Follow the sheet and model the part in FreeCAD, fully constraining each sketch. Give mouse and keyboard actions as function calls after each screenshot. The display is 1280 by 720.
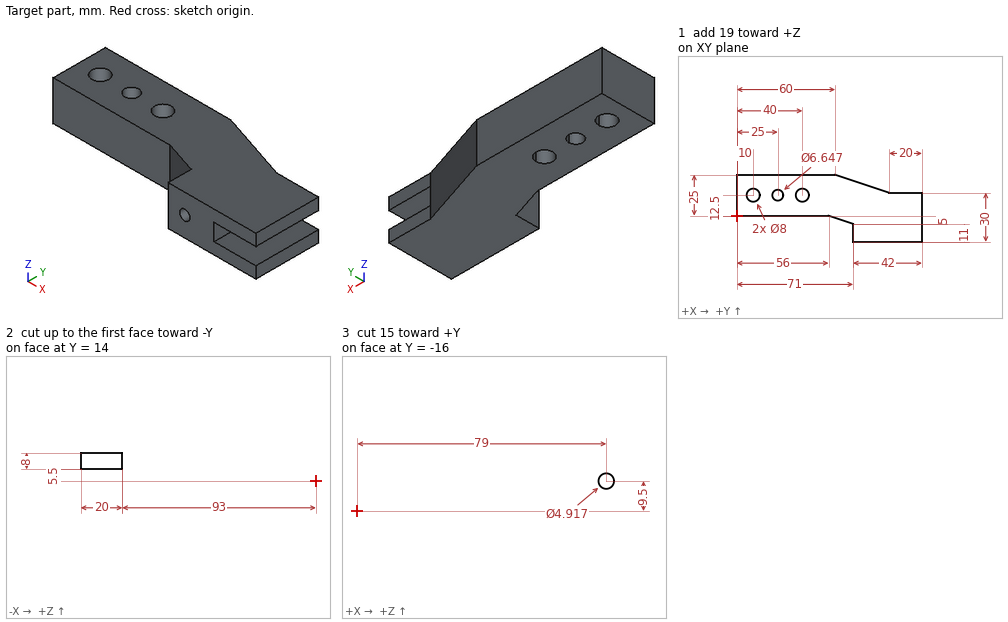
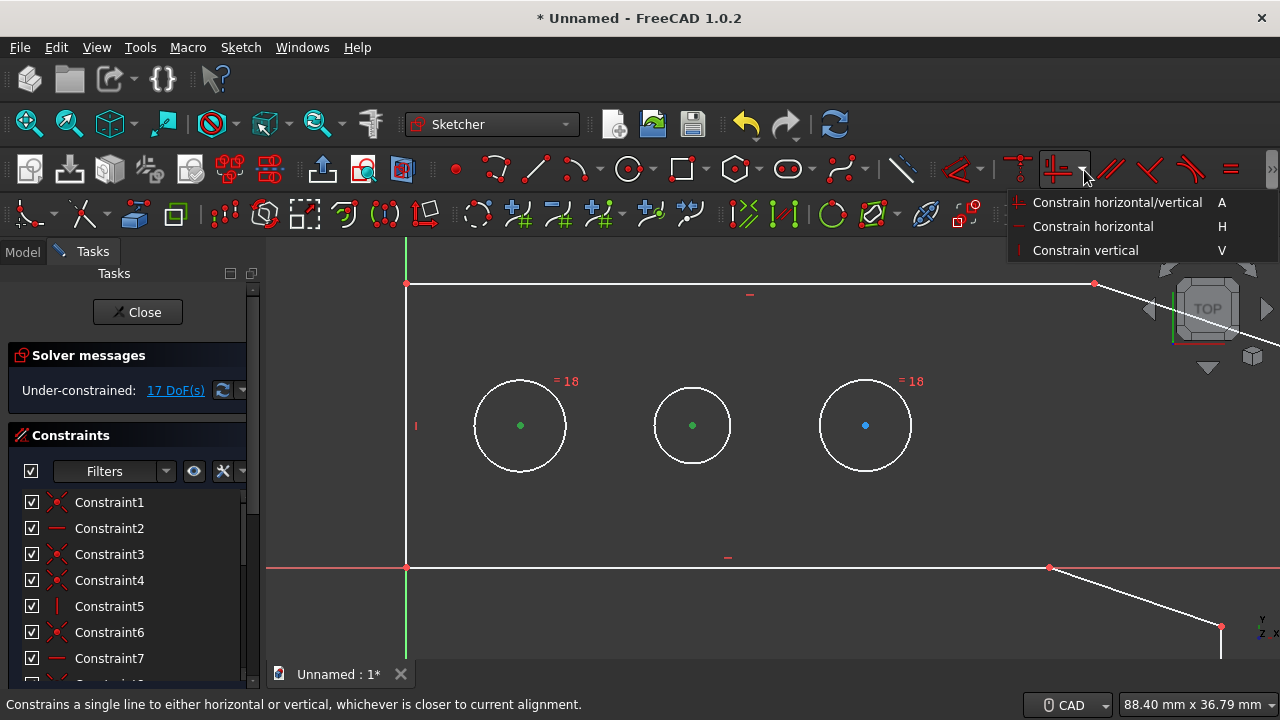
click(1143, 226)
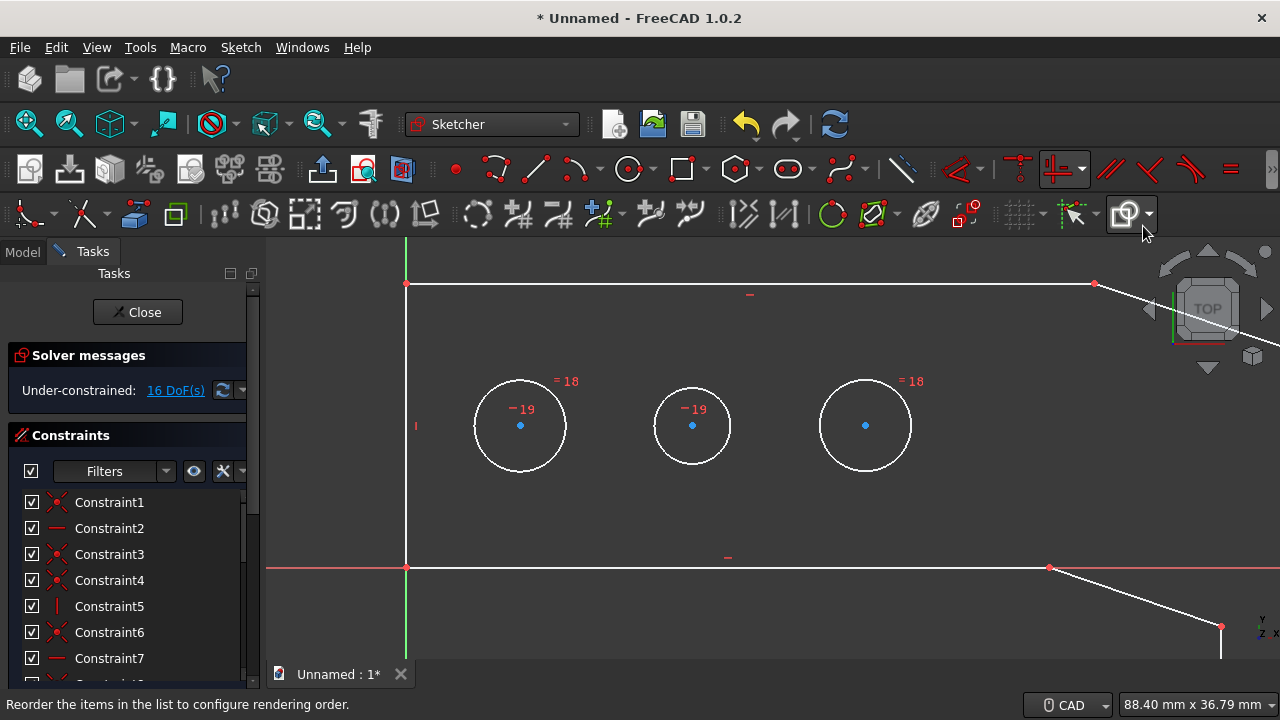
click(692, 426)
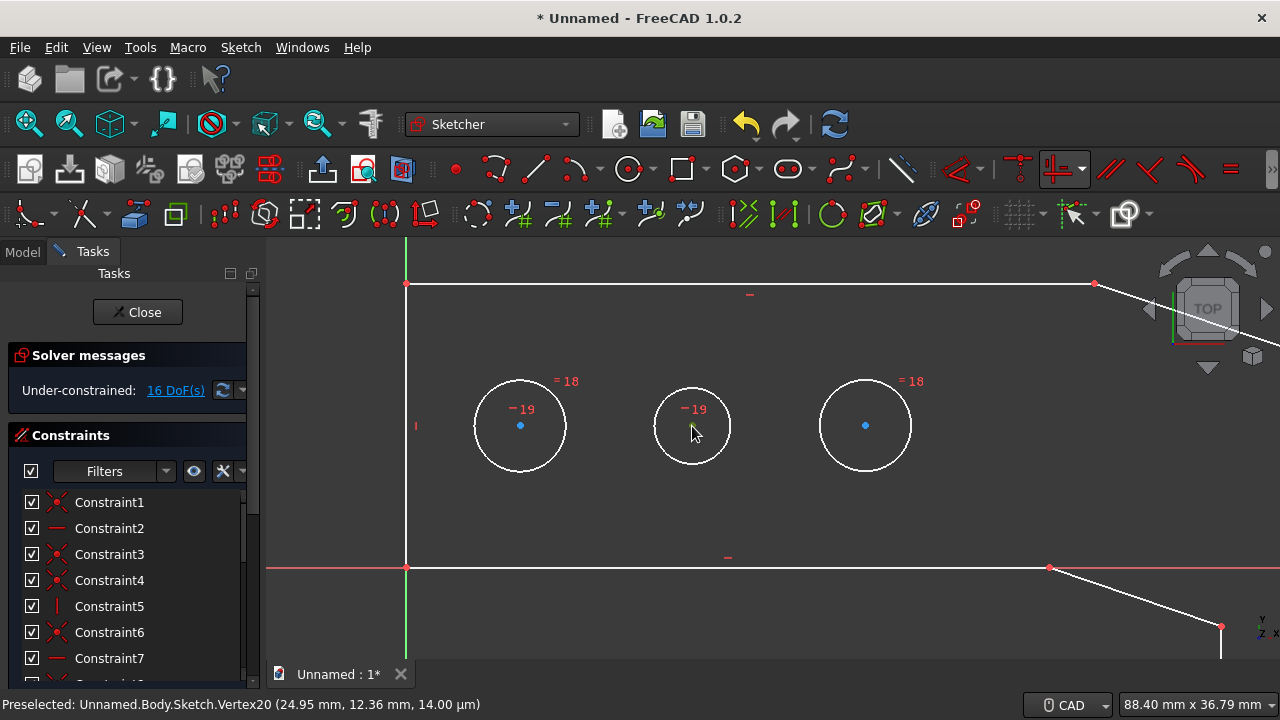
click(865, 426)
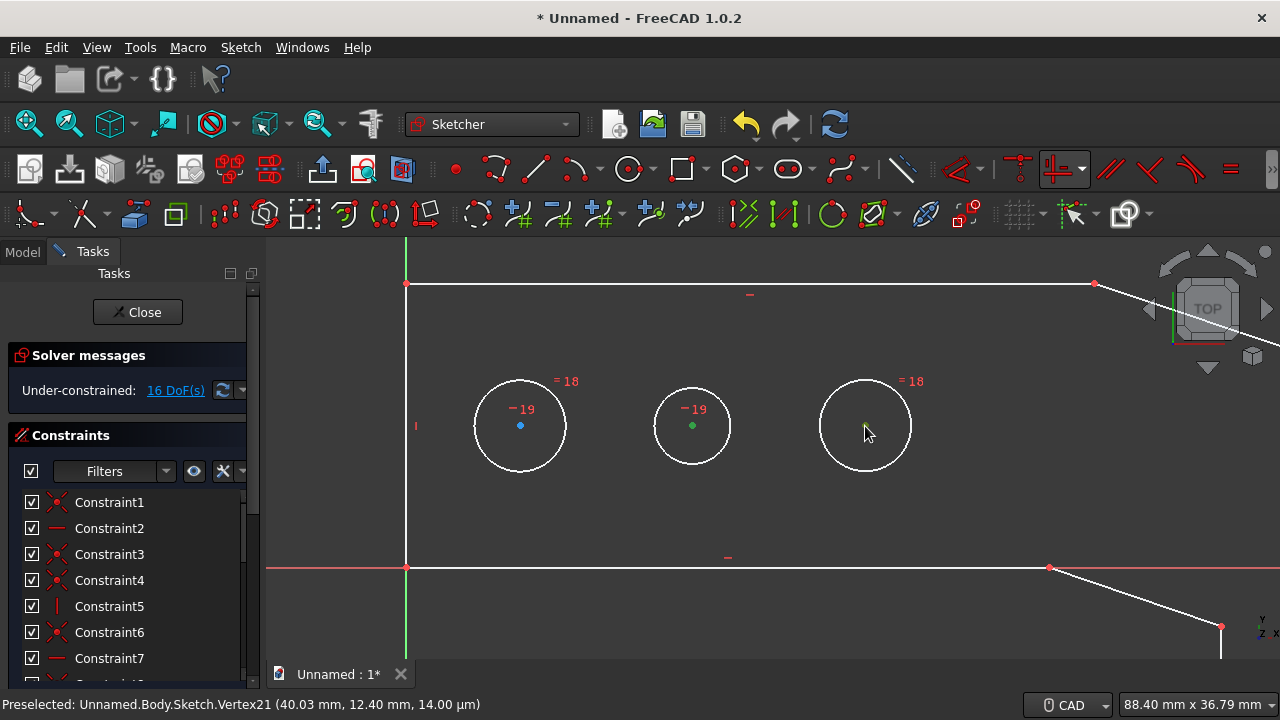
click(1084, 170)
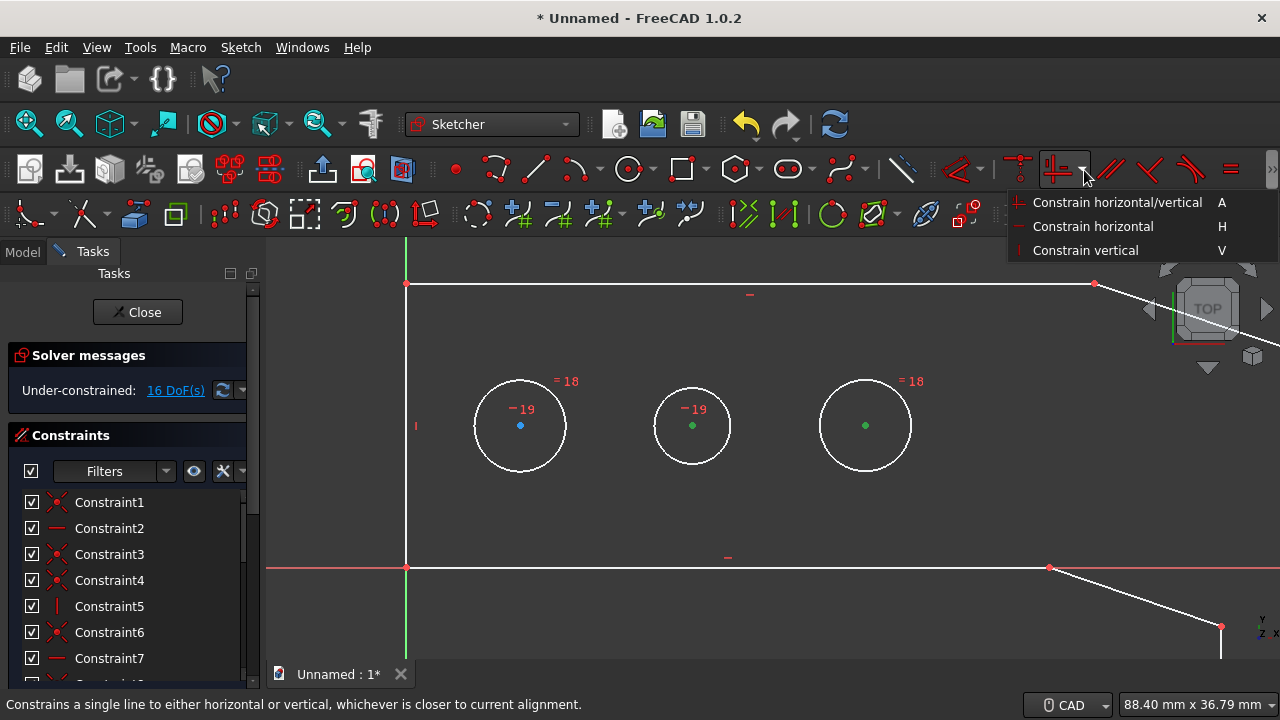
click(1143, 226)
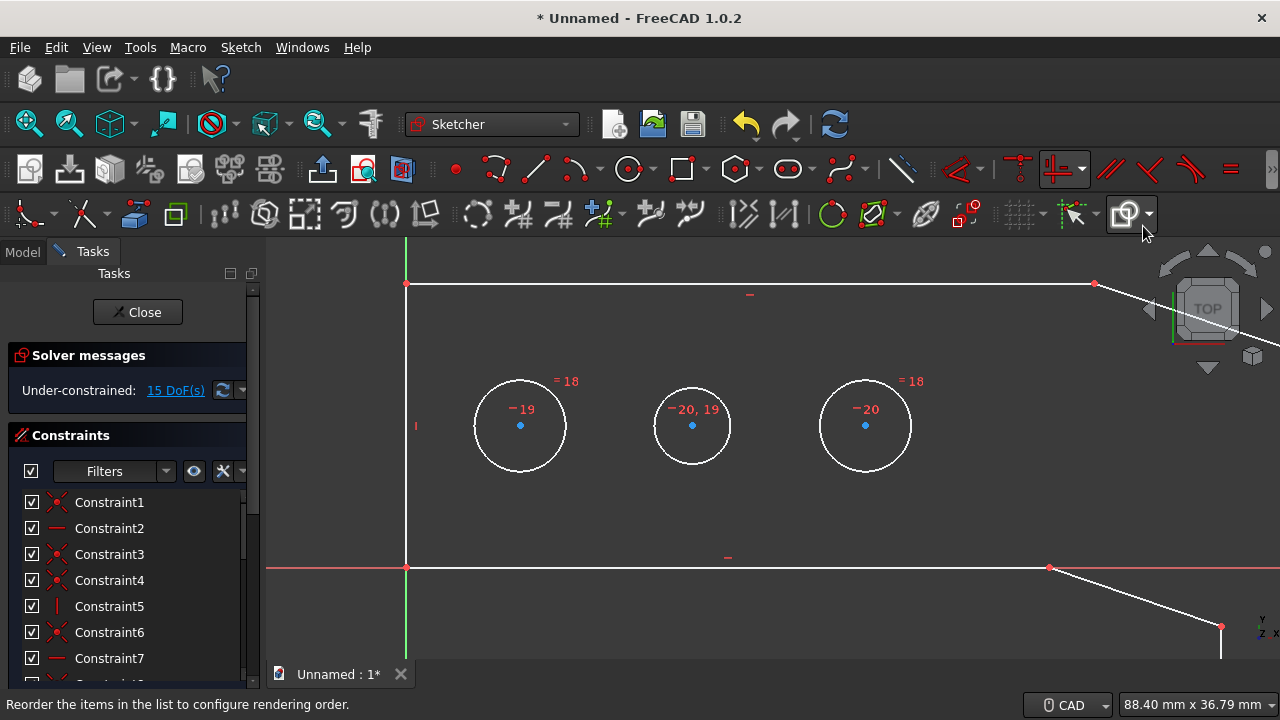
click(956, 170)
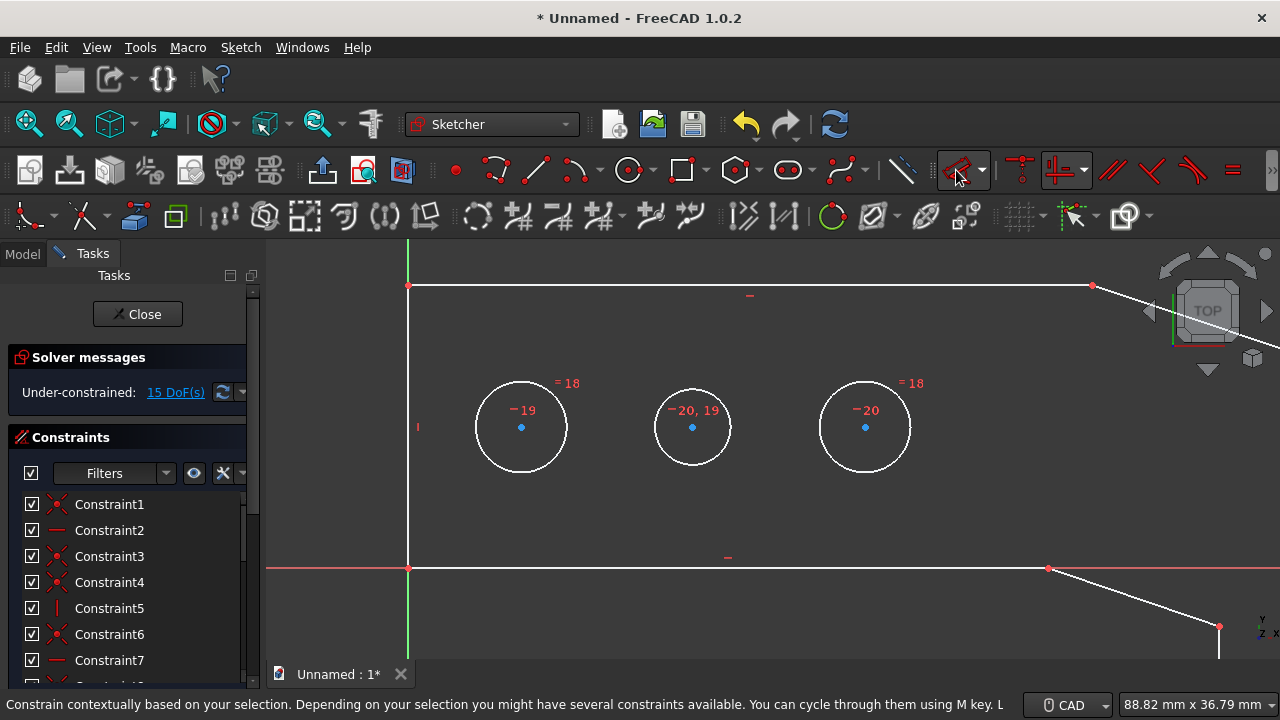
click(553, 395)
click(575, 372)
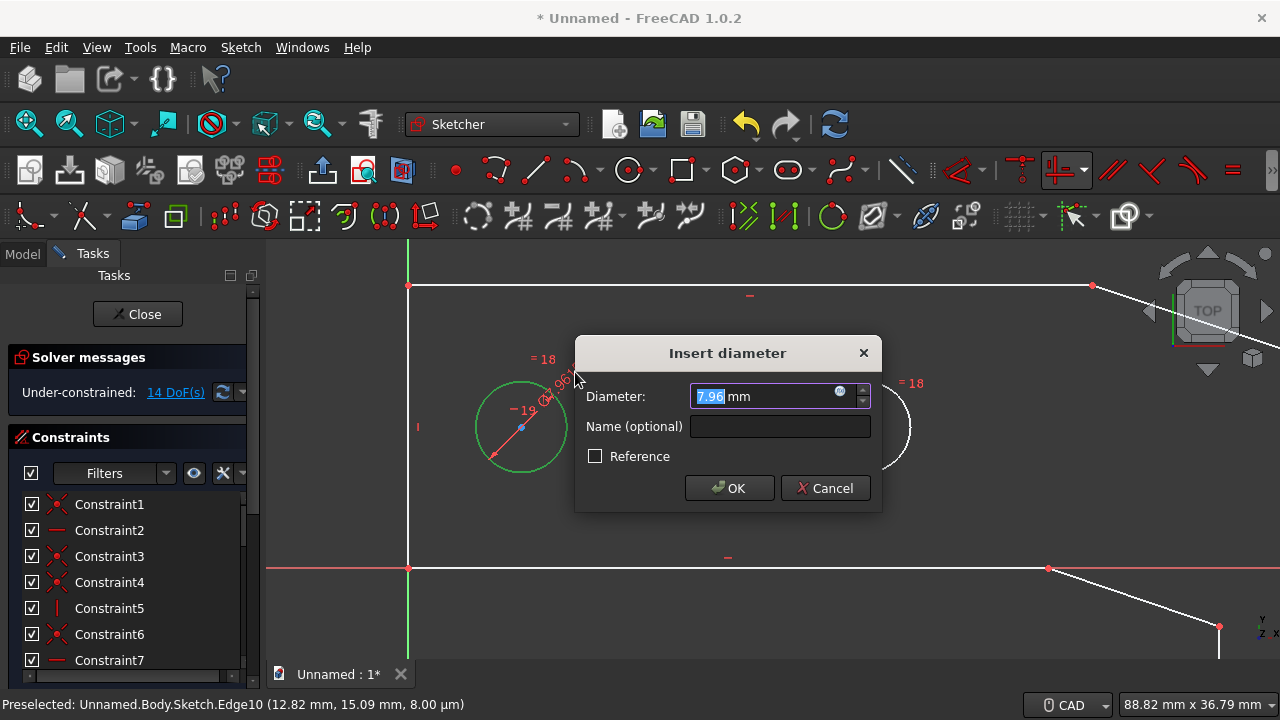
text(8)
key(Return)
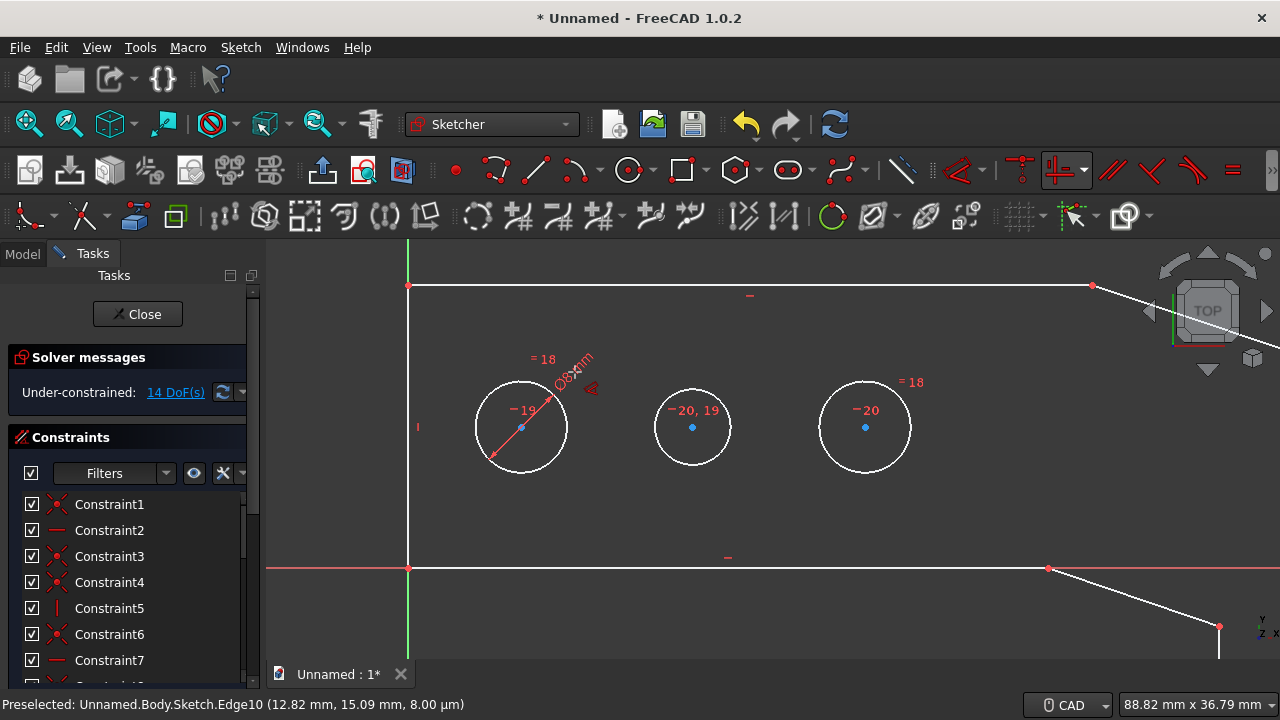
click(719, 400)
click(741, 377)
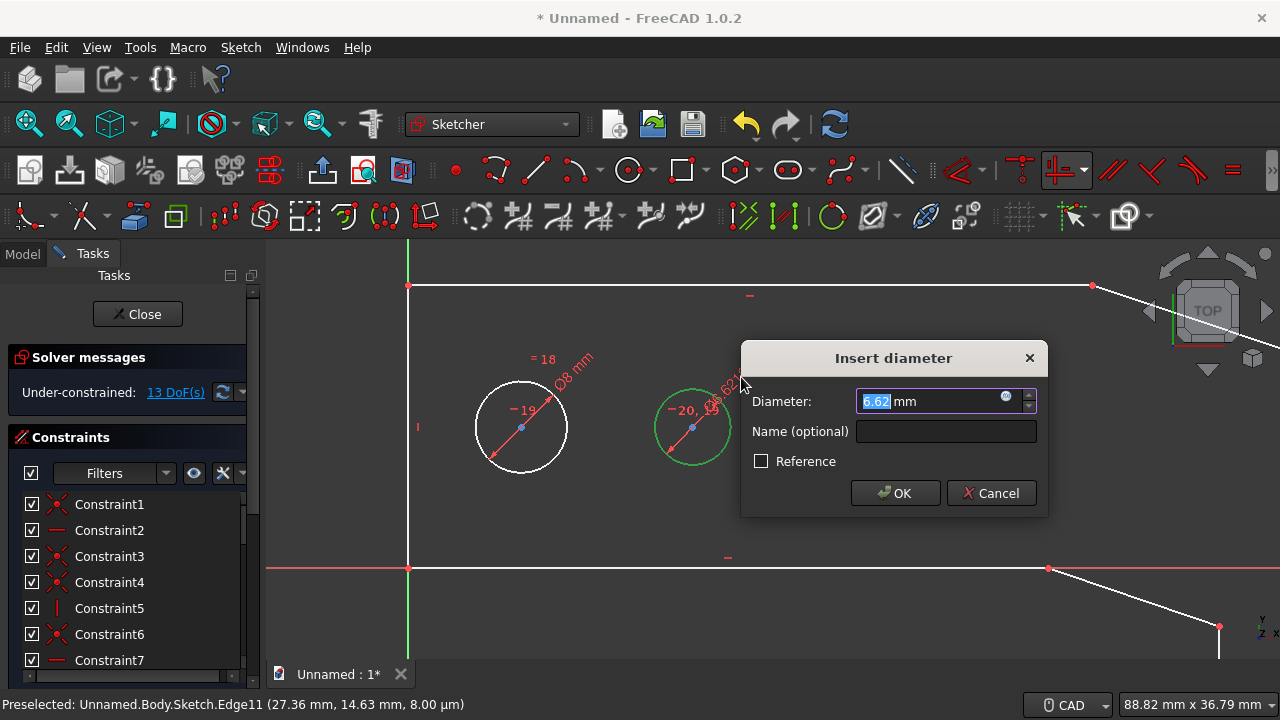
text(6.647)
key(Return)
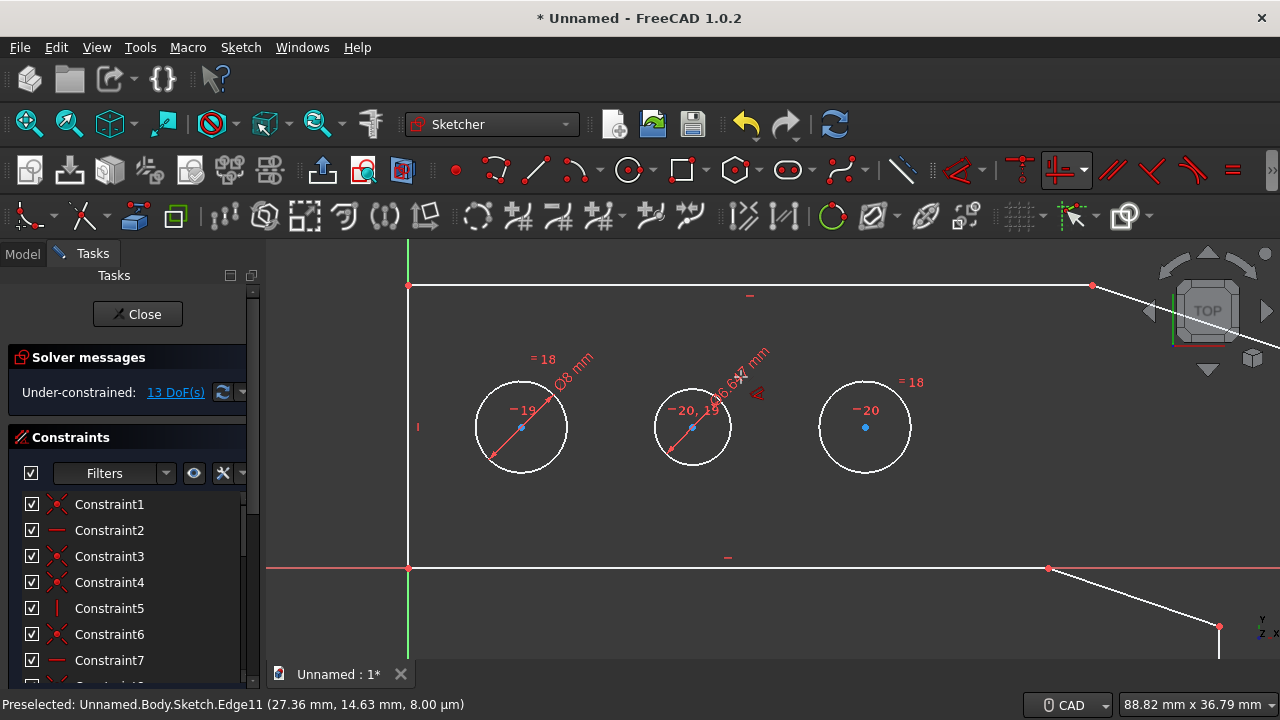
click(600, 568)
click(728, 602)